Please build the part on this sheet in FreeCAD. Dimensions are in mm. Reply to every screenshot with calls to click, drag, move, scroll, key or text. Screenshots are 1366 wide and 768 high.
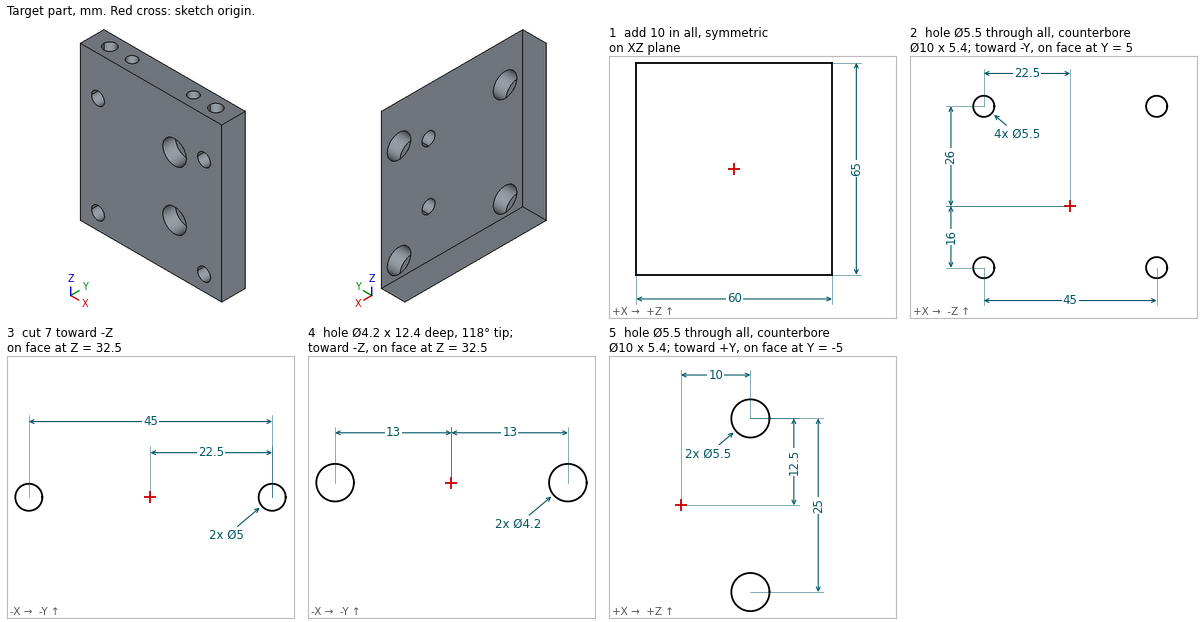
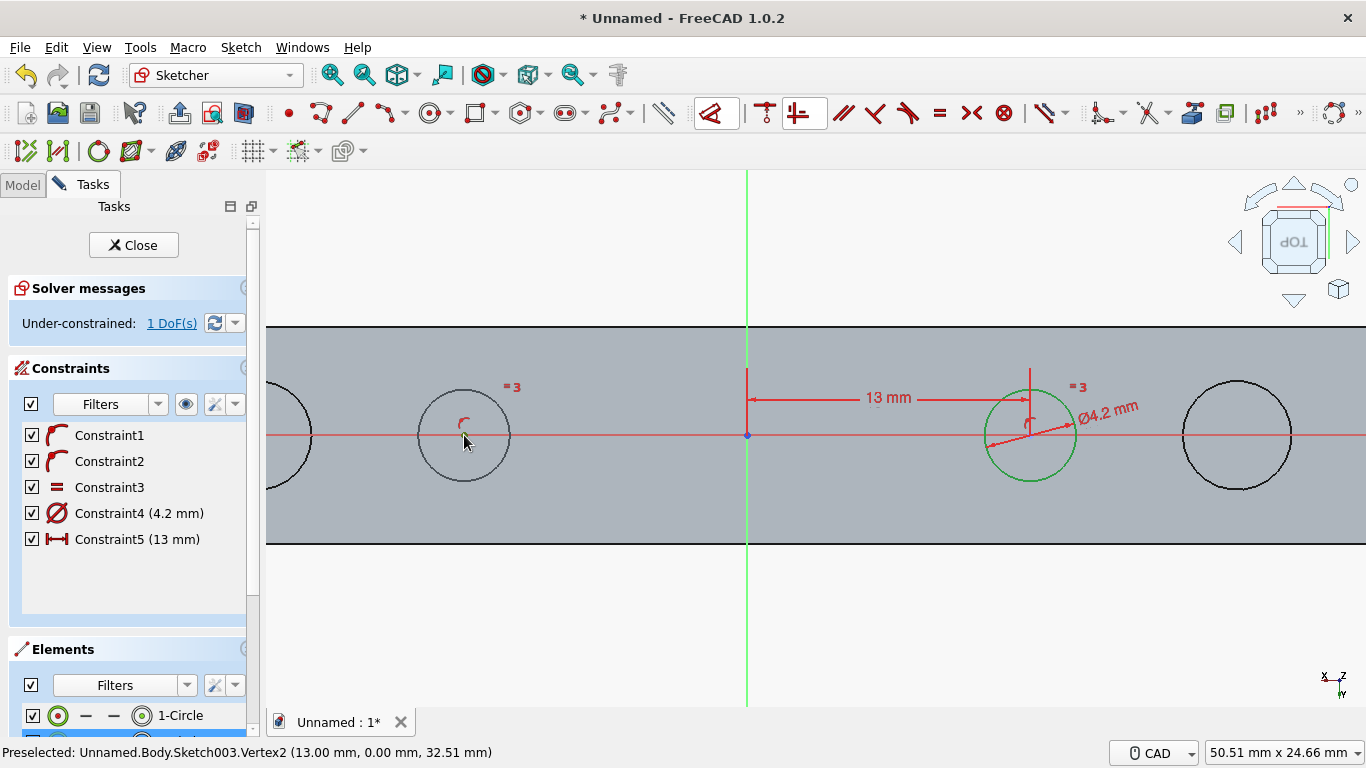
click(734, 114)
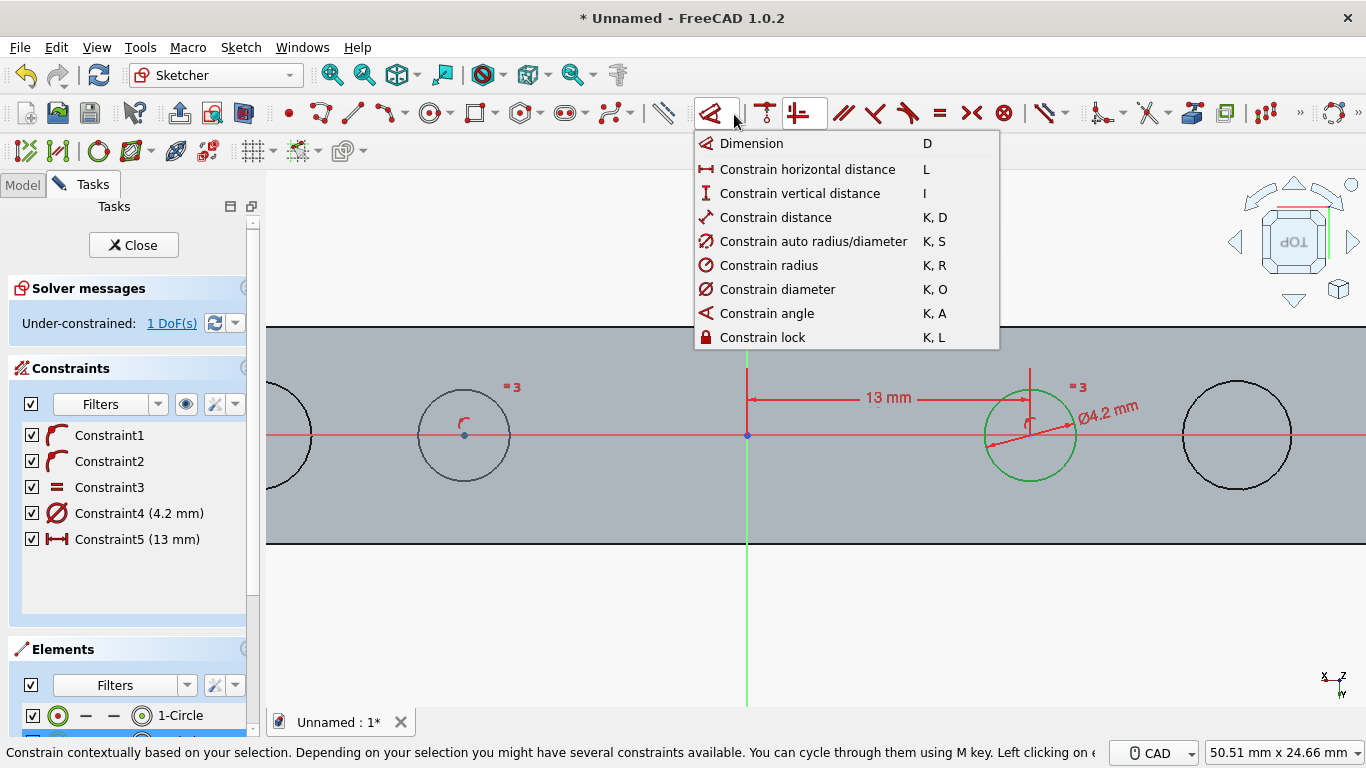
click(847, 169)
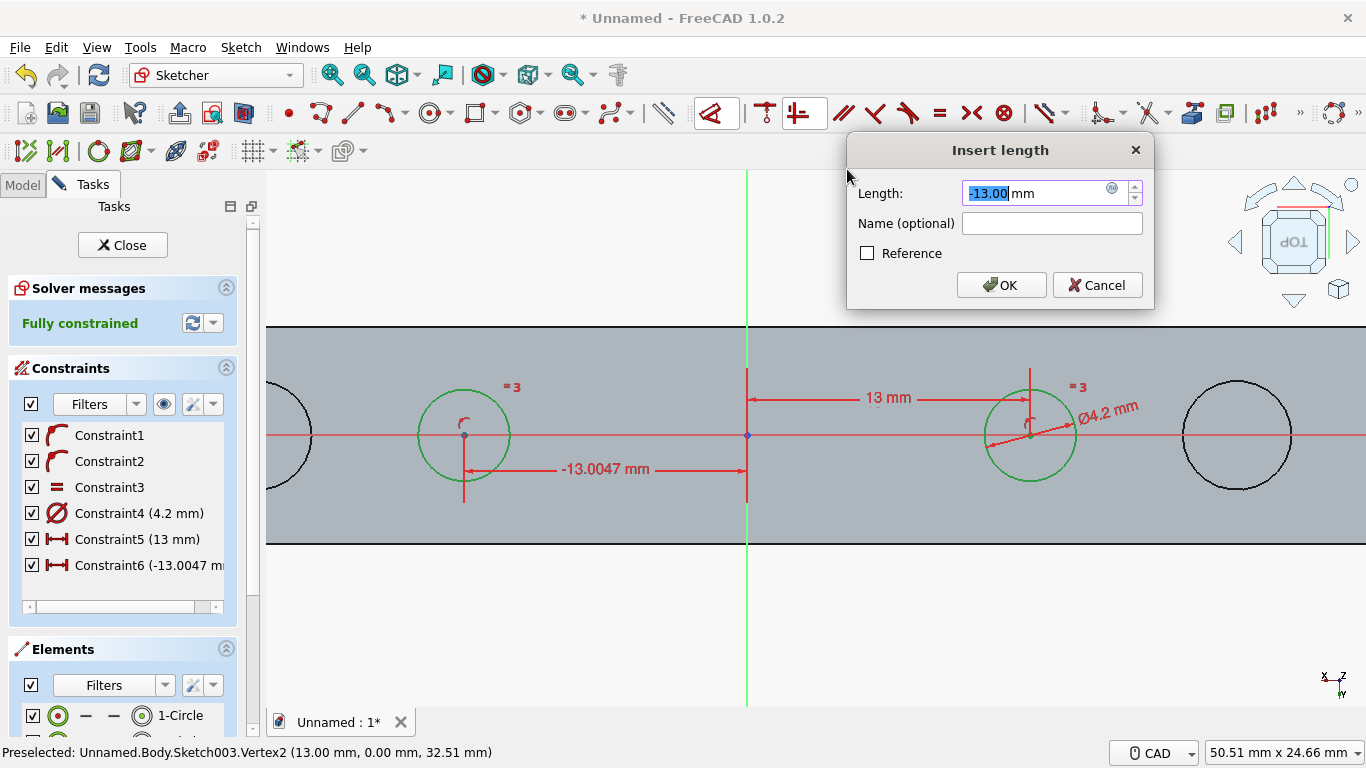
text(-13)
key(Return)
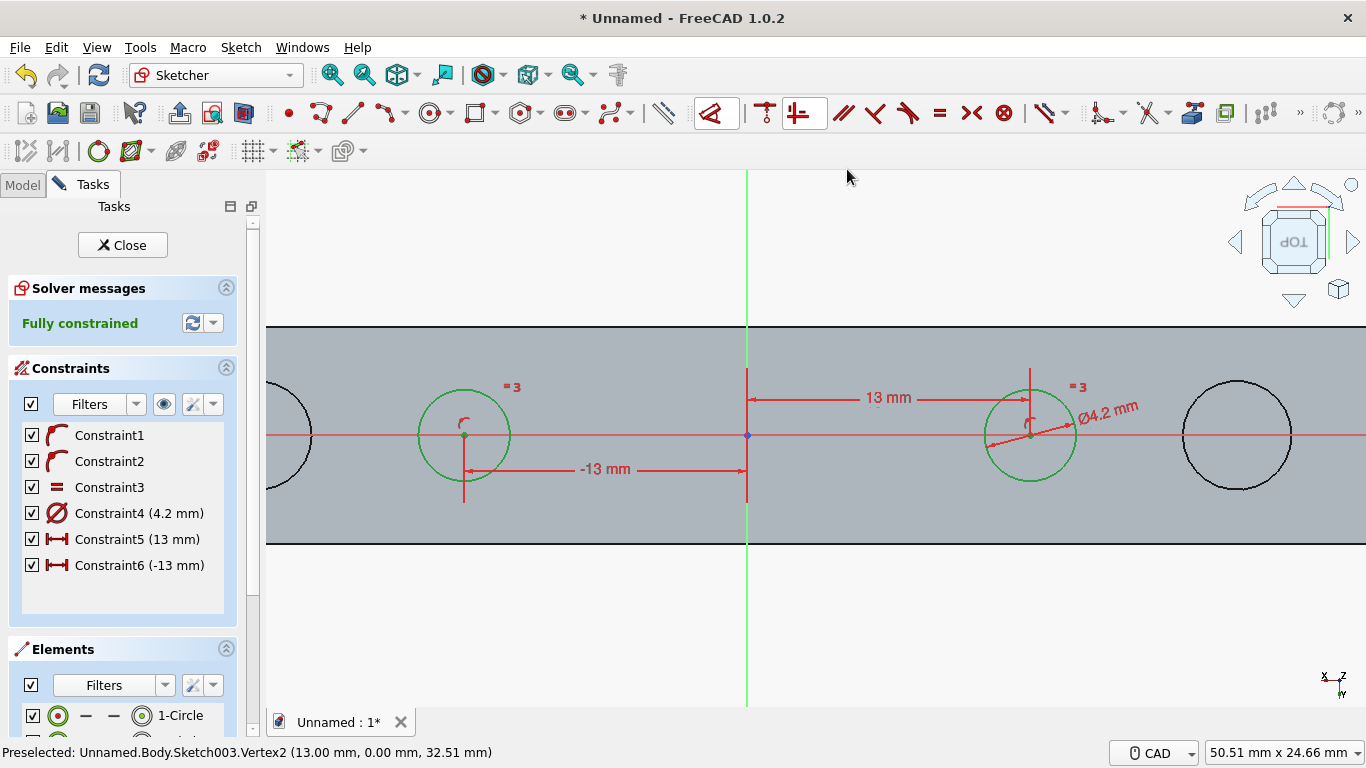
click(123, 245)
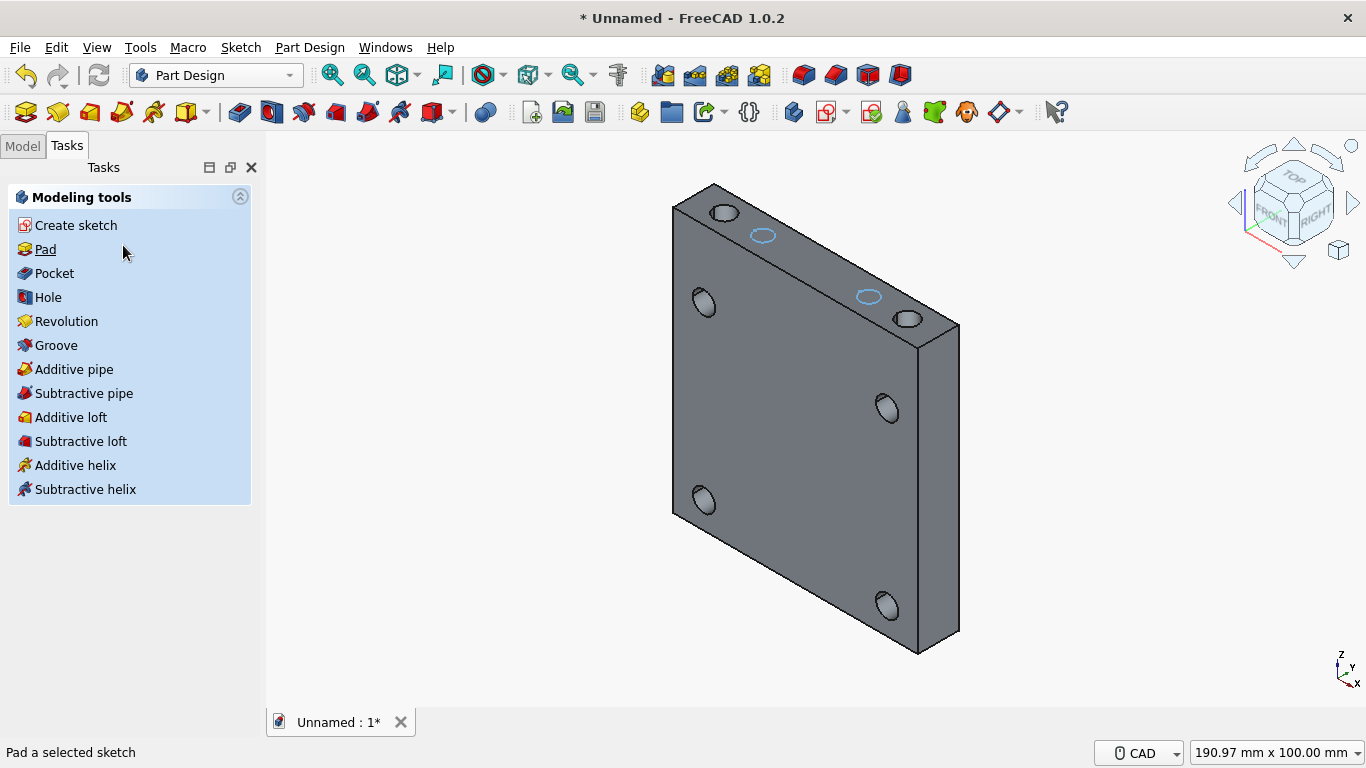
click(272, 112)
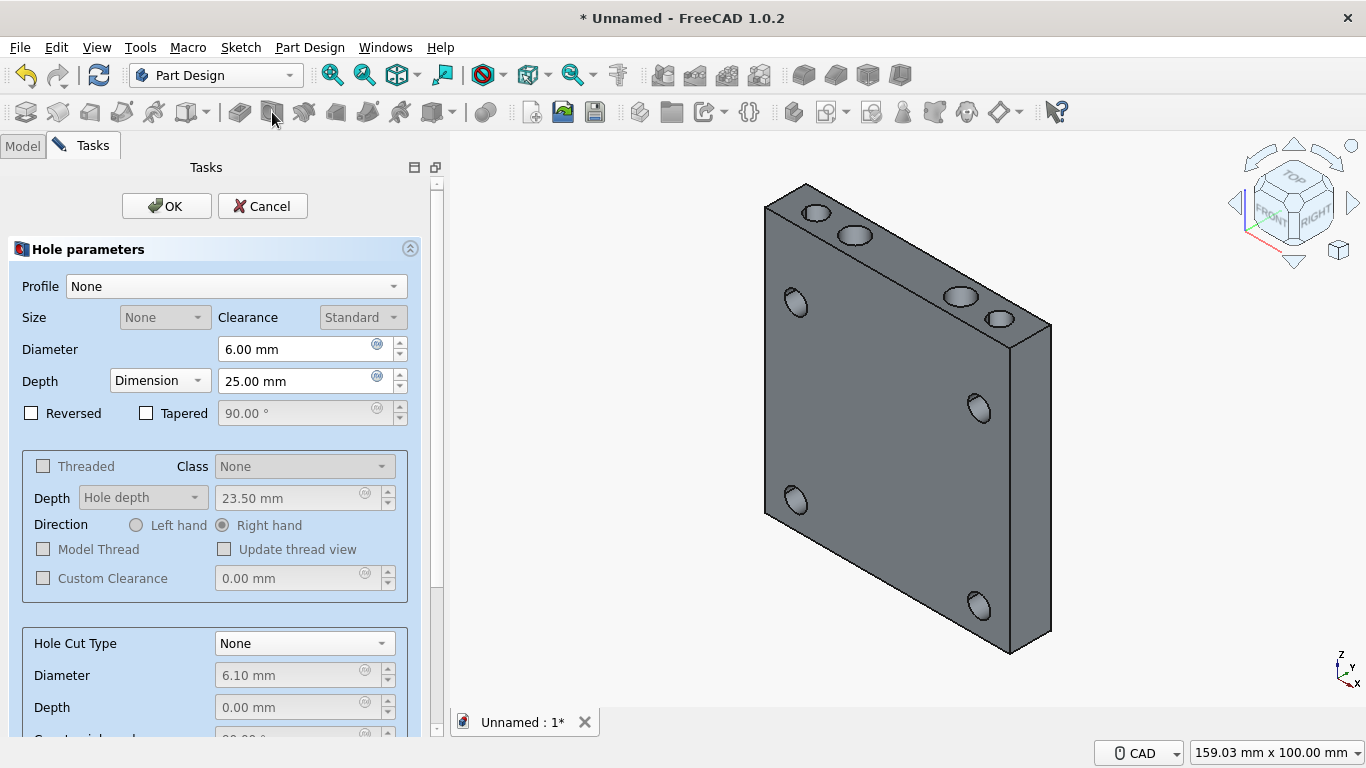
triple_click(305, 349)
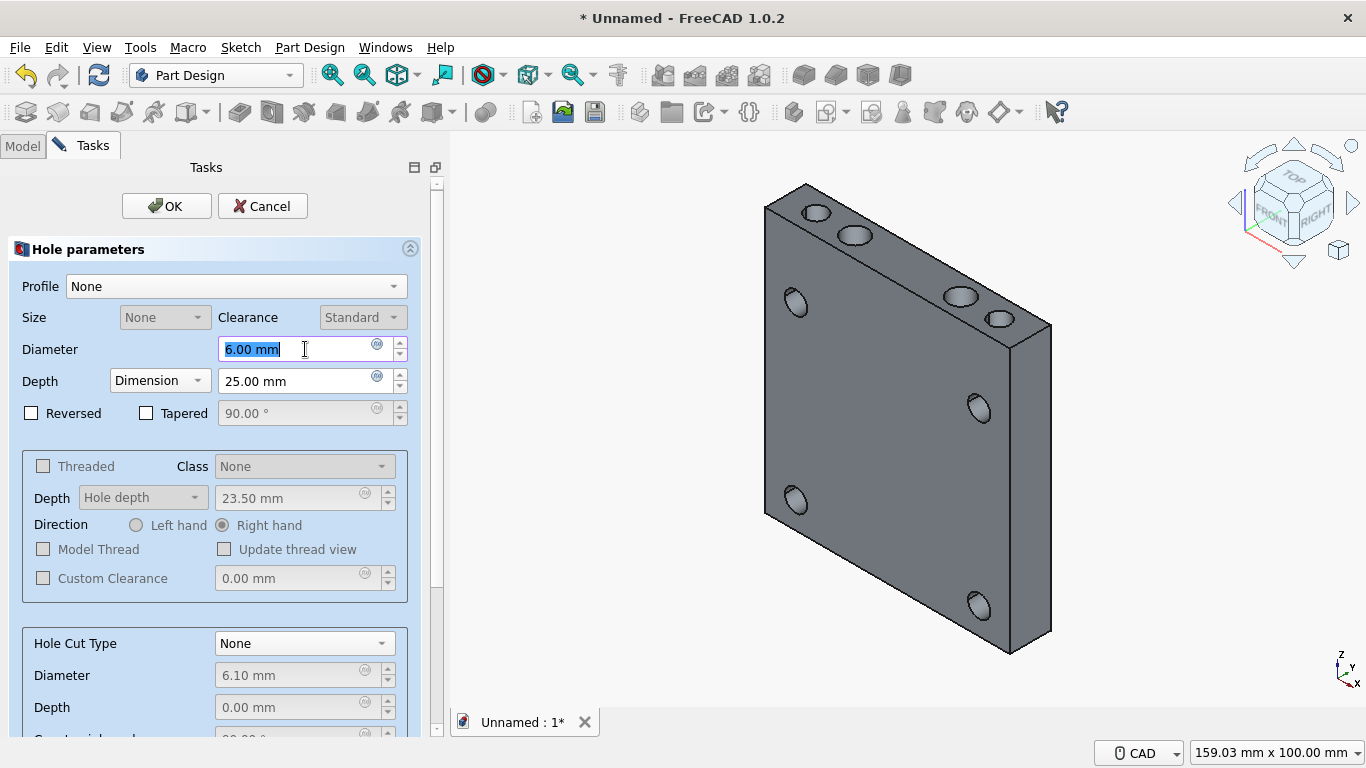
text(4.2)
key(Tab)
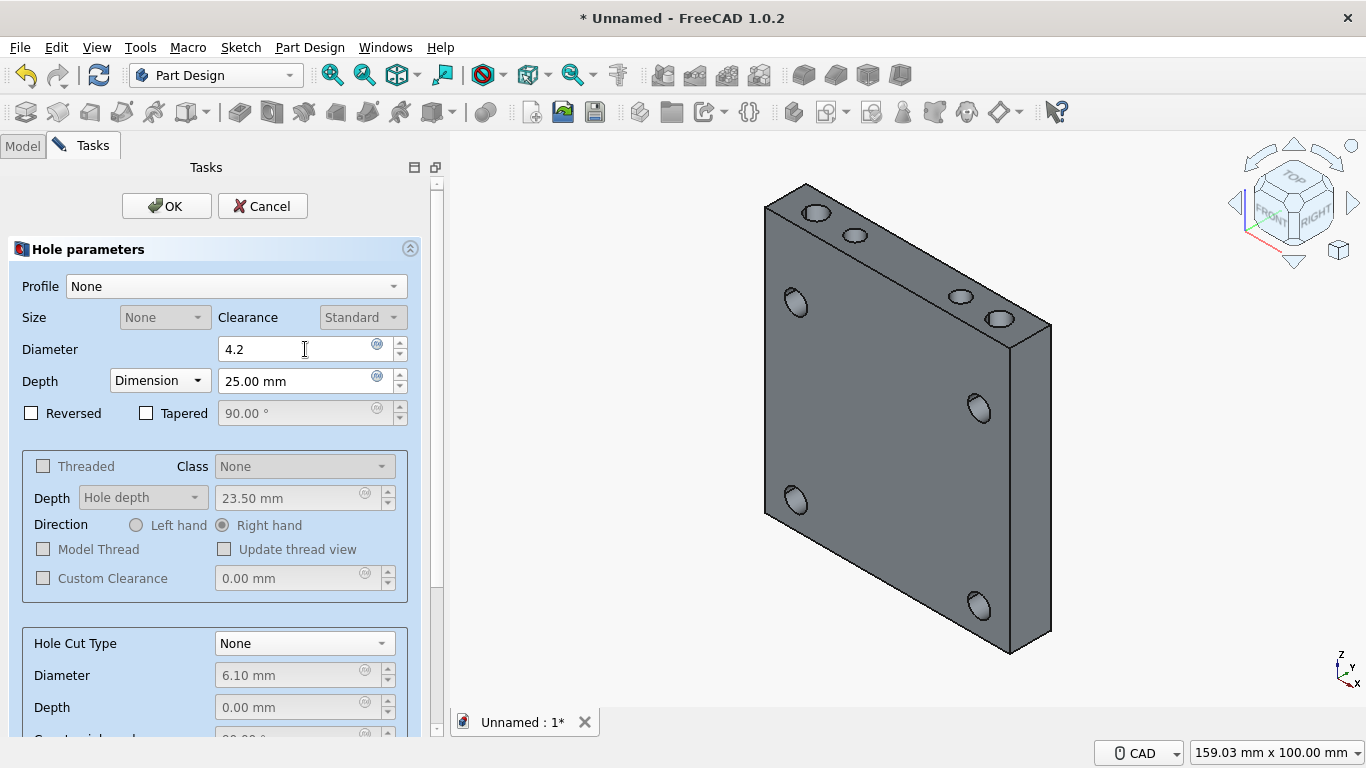
triple_click(305, 381)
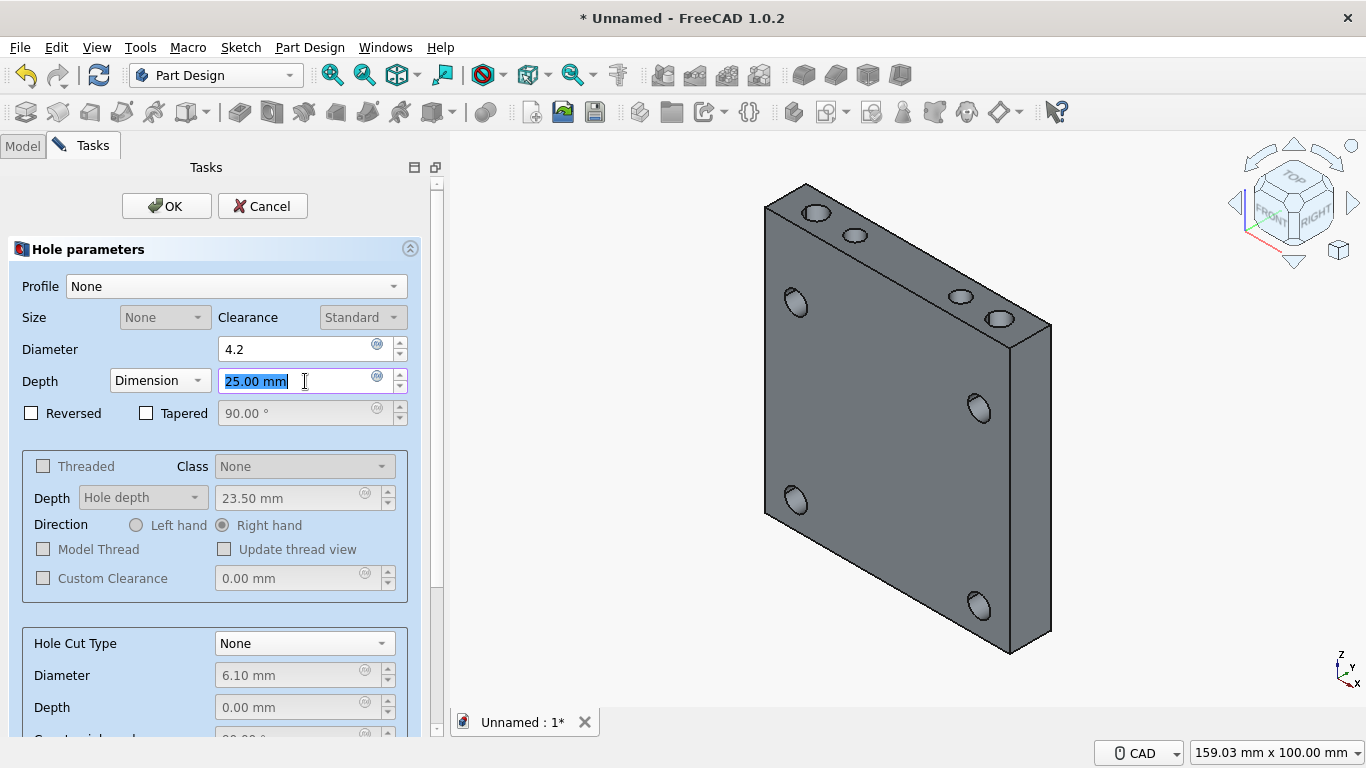
text(12.4)
key(Tab)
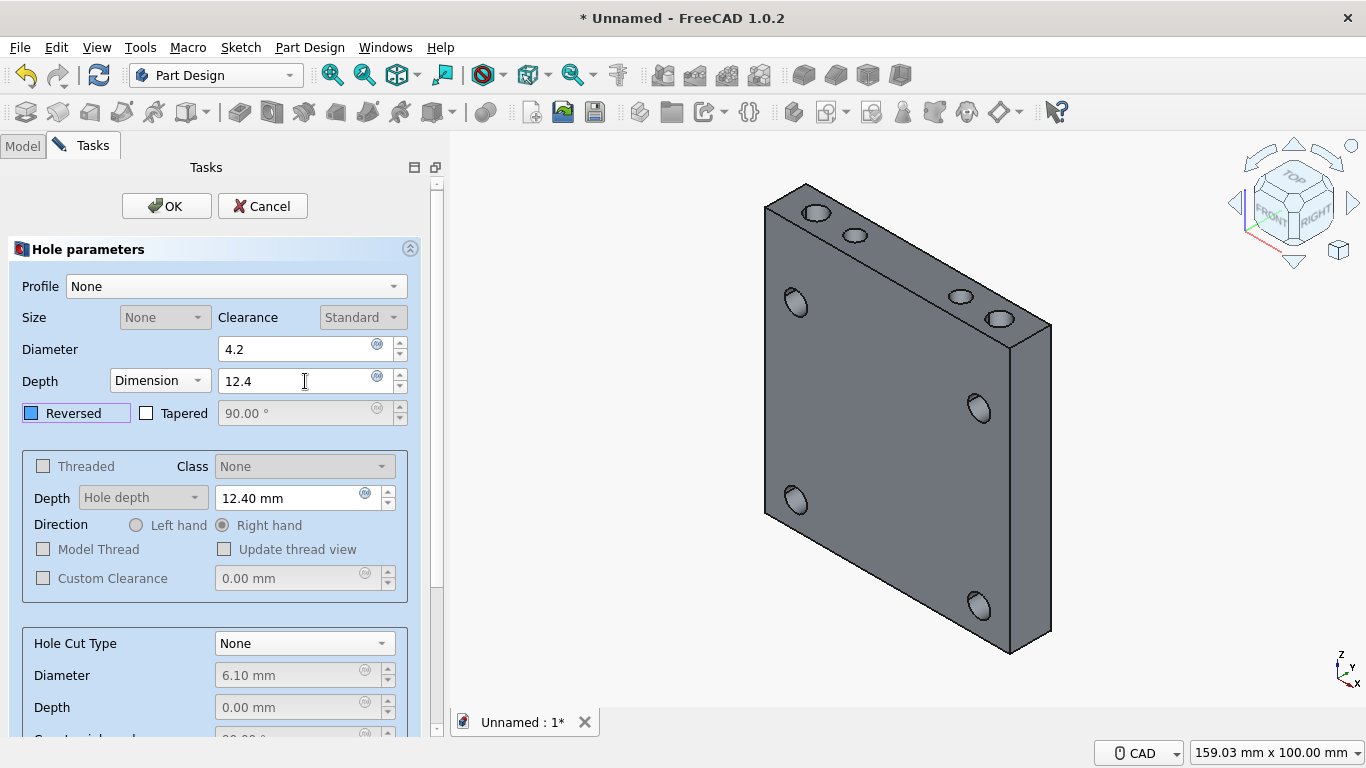
click(167, 206)